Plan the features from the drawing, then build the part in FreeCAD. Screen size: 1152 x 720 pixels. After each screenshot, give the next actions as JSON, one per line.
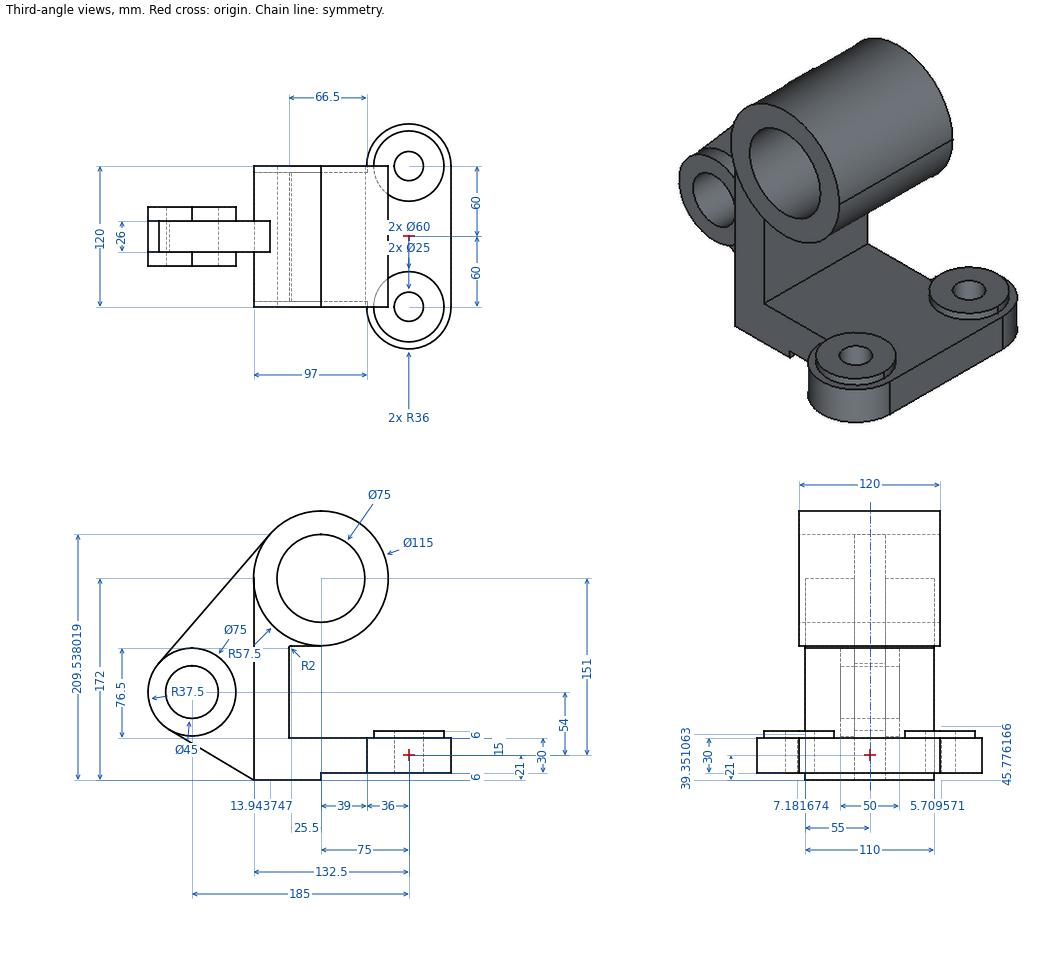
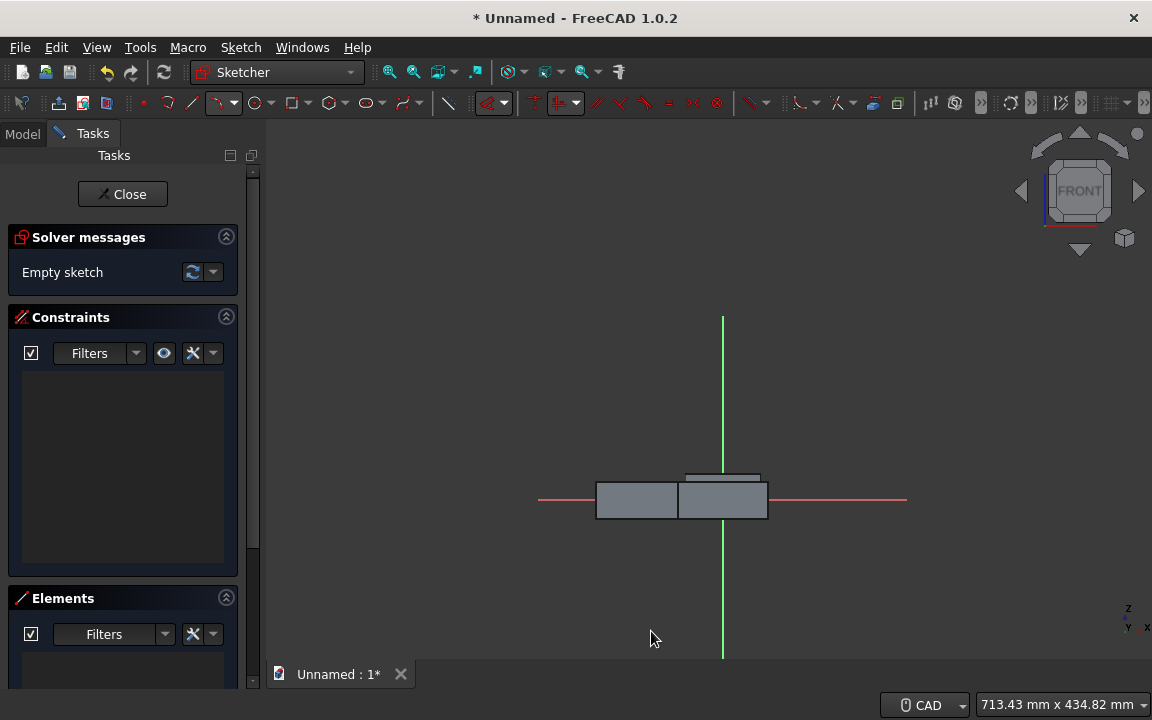
{"action": "left_click", "coordinate": [256, 104]}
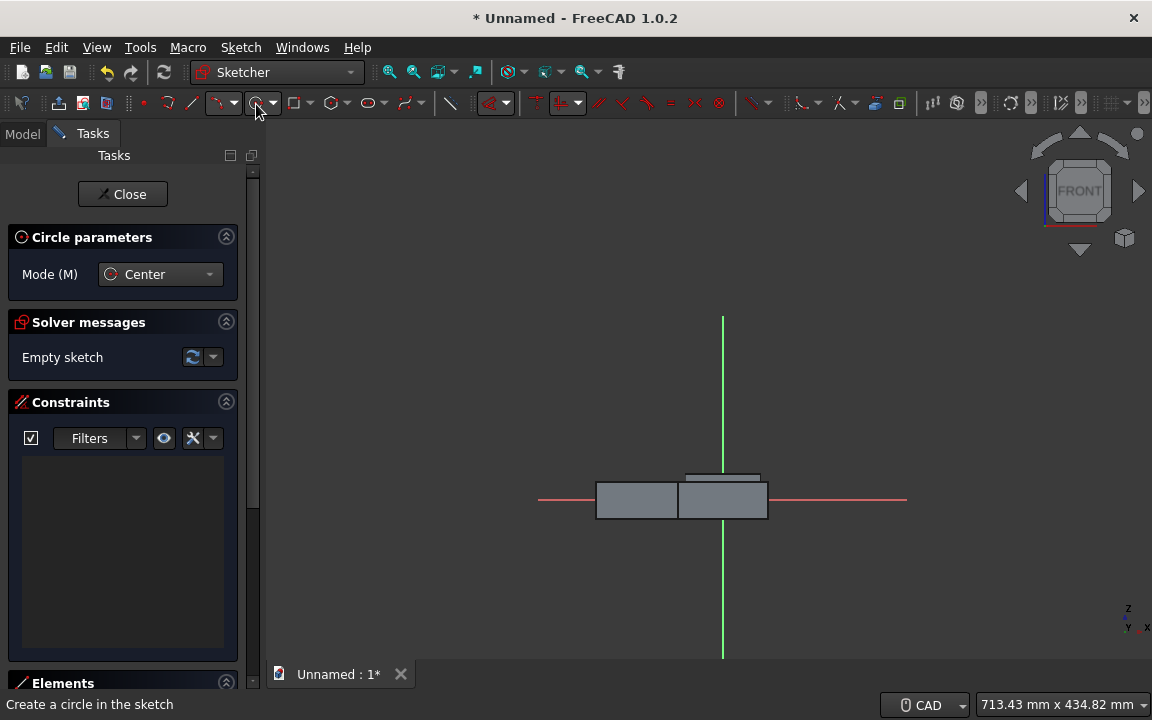
{"action": "left_click", "coordinate": [630, 313]}
{"action": "left_click", "coordinate": [680, 262]}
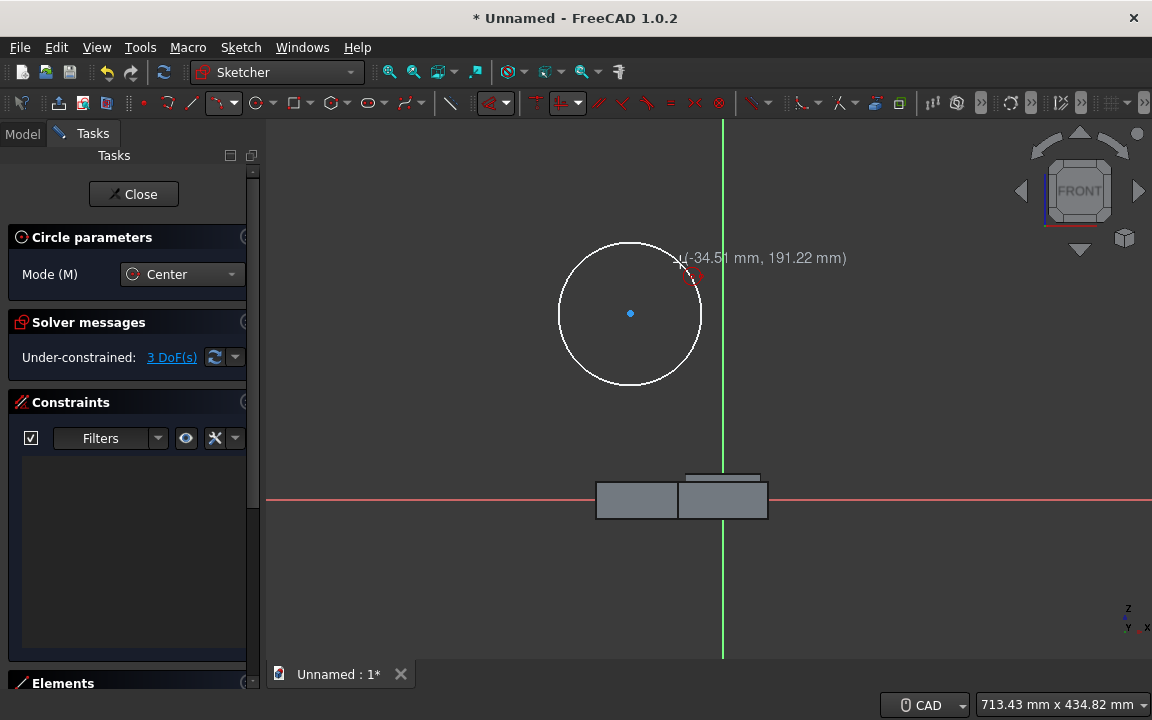
{"action": "left_click", "coordinate": [630, 314]}
{"action": "left_click", "coordinate": [663, 280]}
{"action": "key", "text": "Escape"}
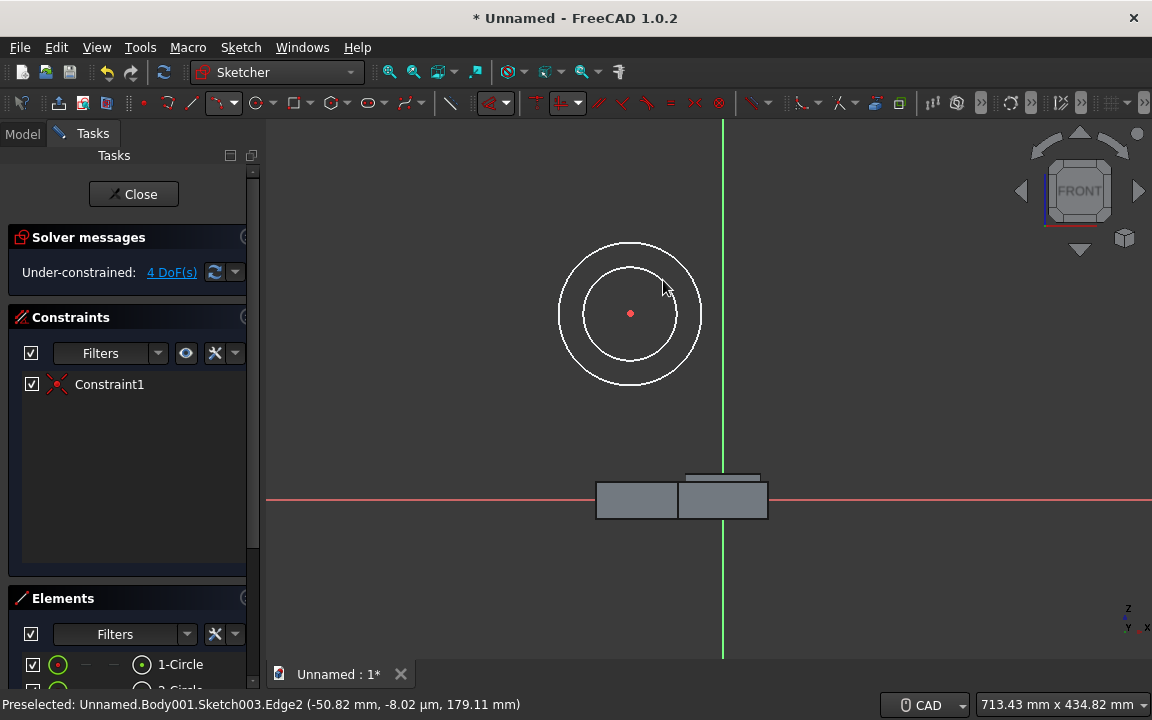
{"action": "left_click", "coordinate": [680, 263]}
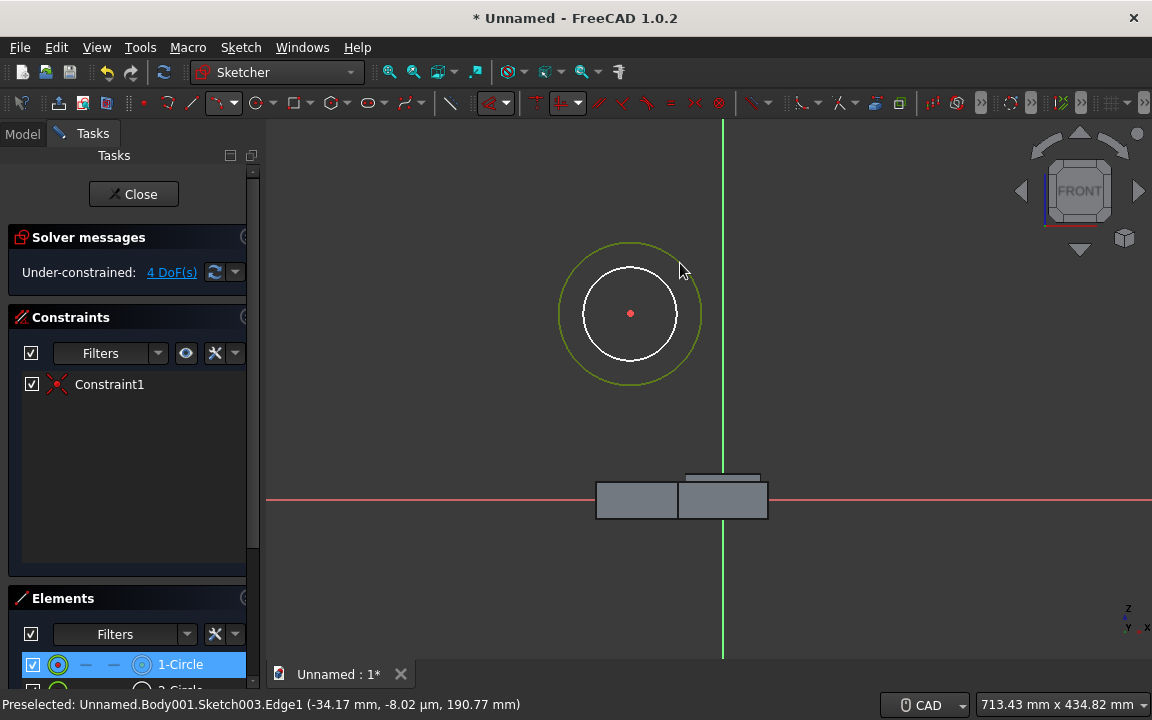
{"action": "key", "text": "k o"}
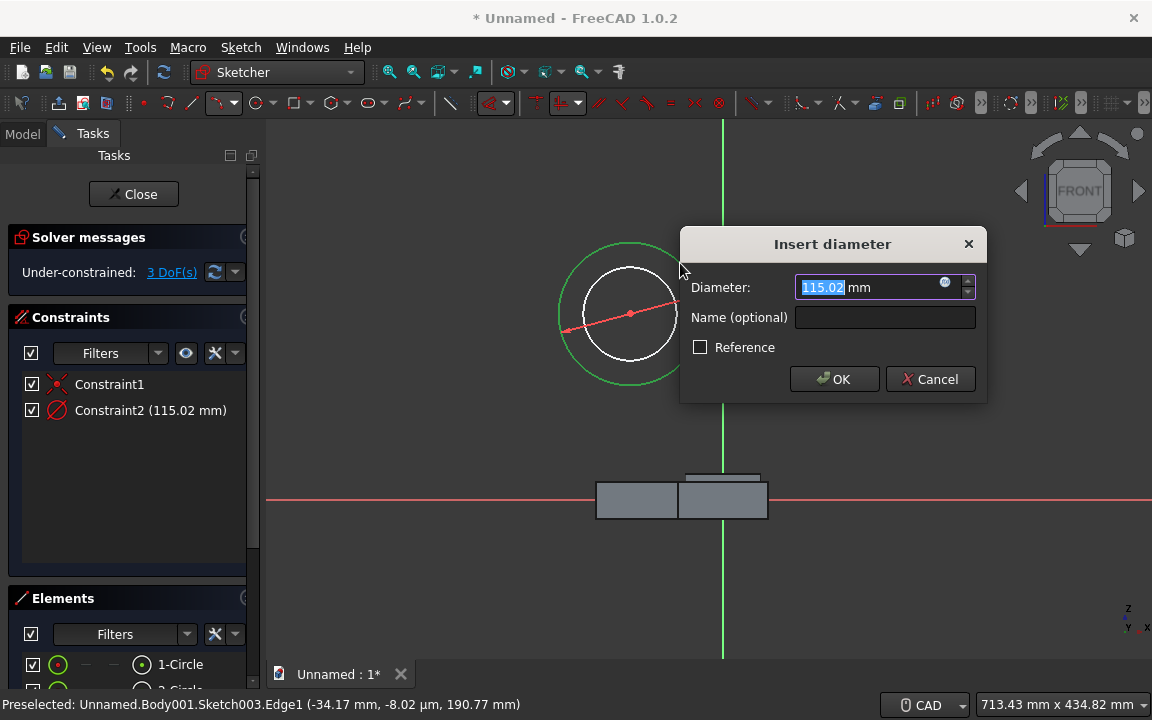
{"action": "type", "text": "115"}
{"action": "key", "text": "Return"}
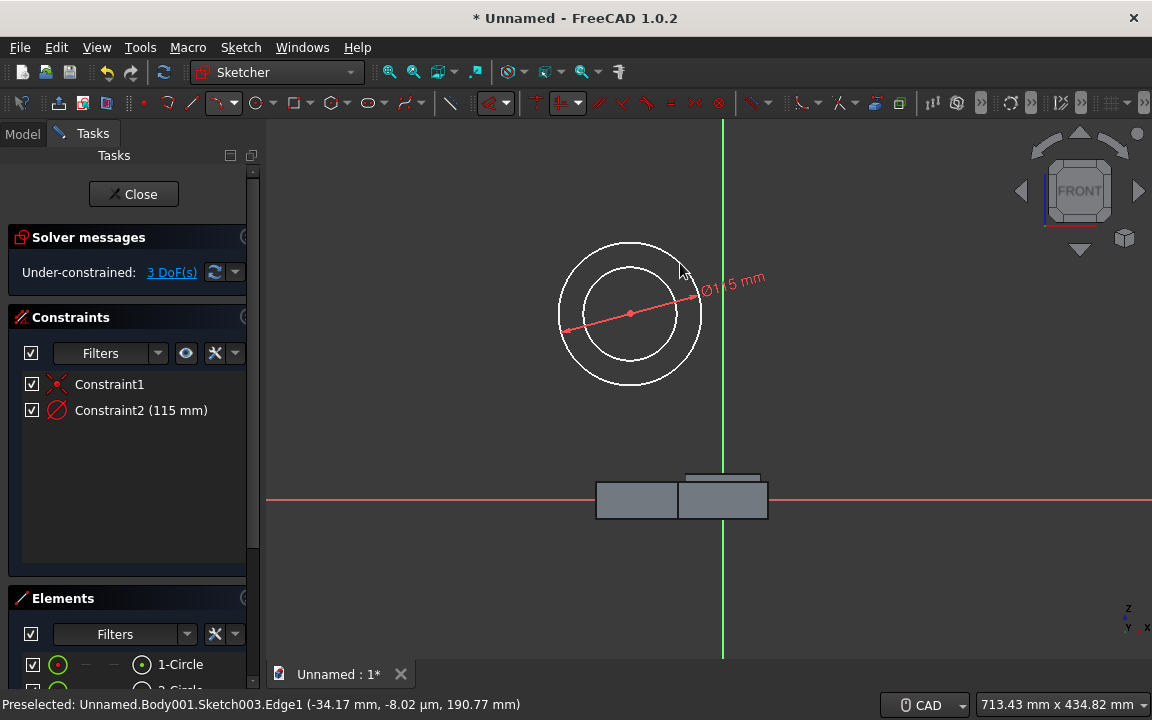
{"action": "left_click", "coordinate": [663, 281]}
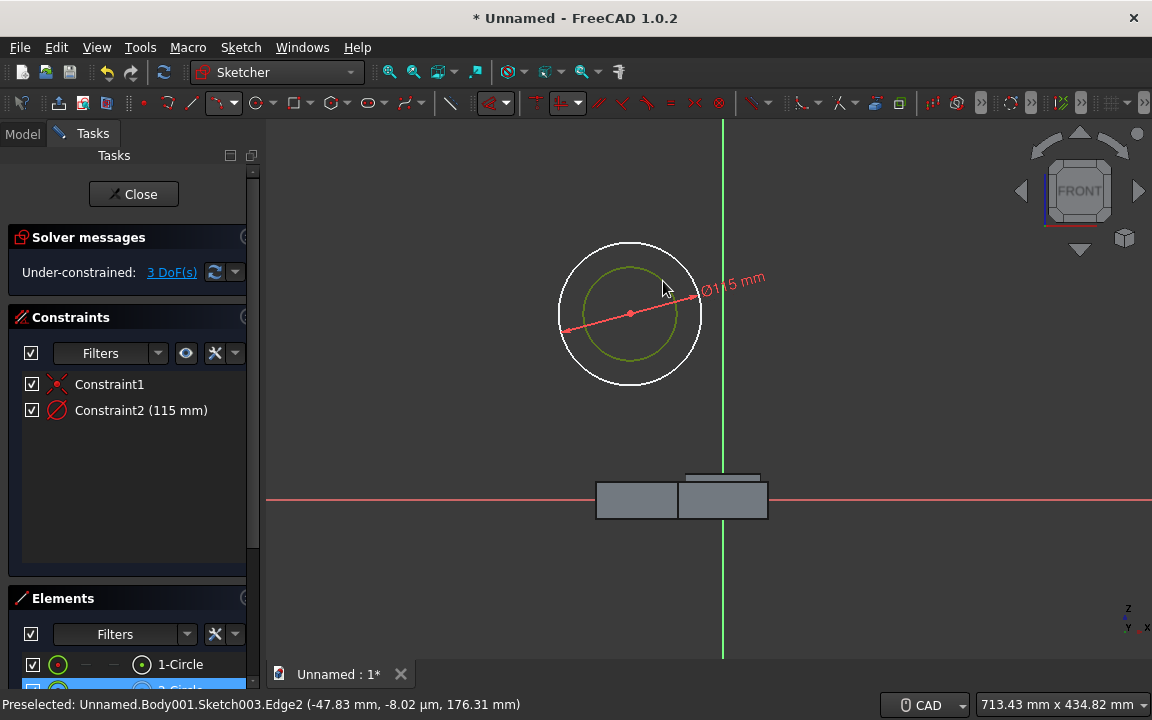
{"action": "key", "text": "k o"}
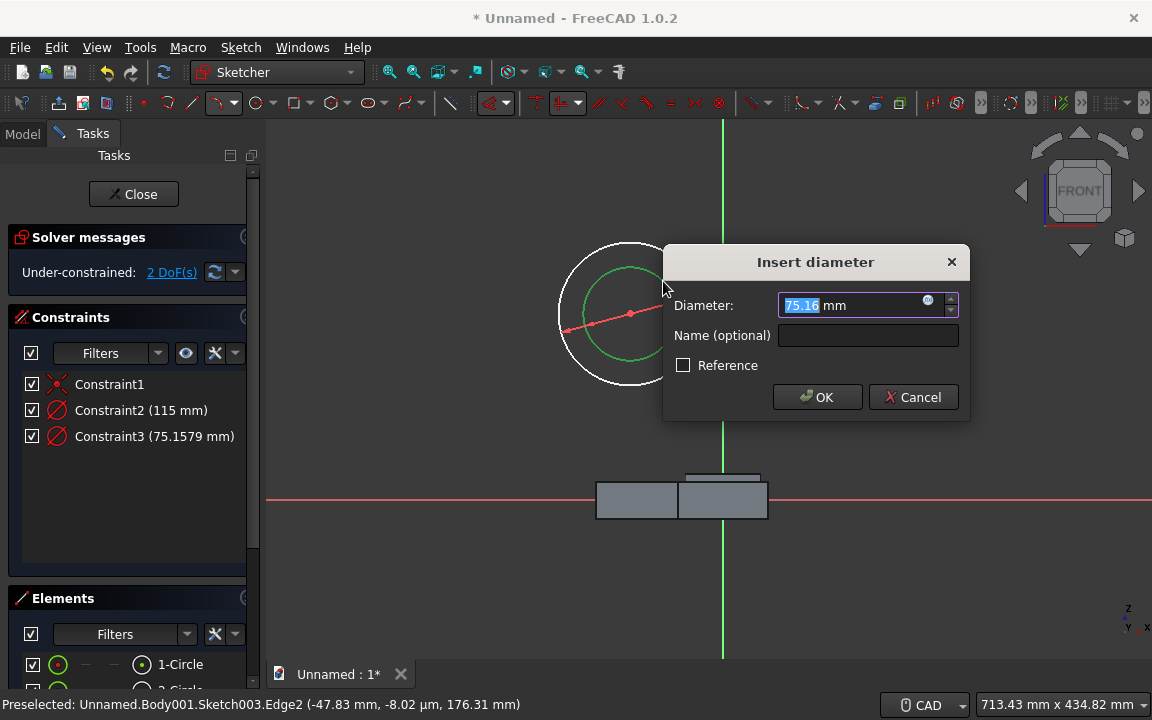
{"action": "type", "text": "75"}
{"action": "key", "text": "Return"}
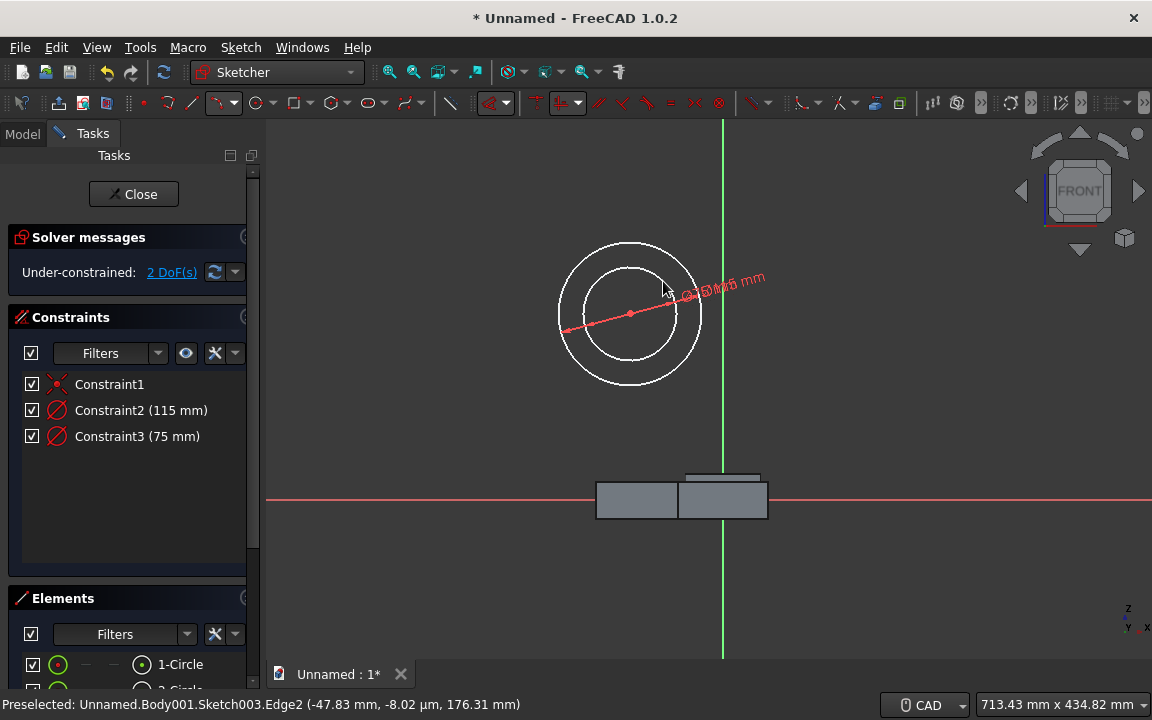
{"action": "left_click", "coordinate": [630, 314]}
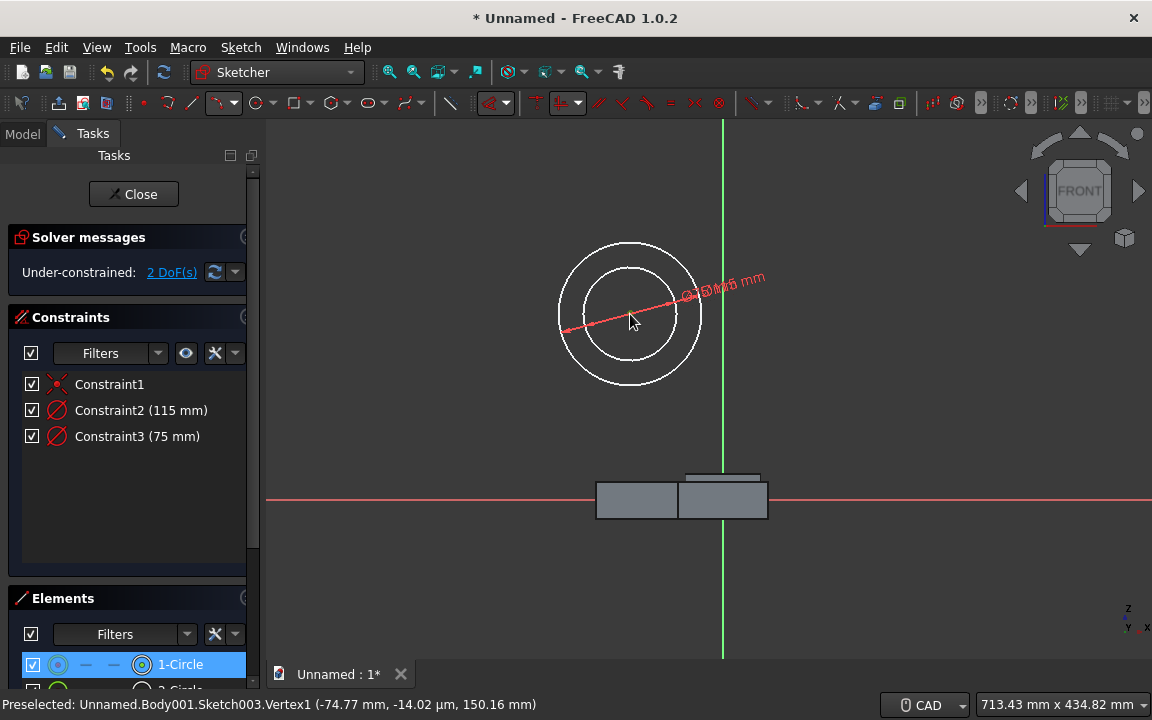
{"action": "key", "text": "l"}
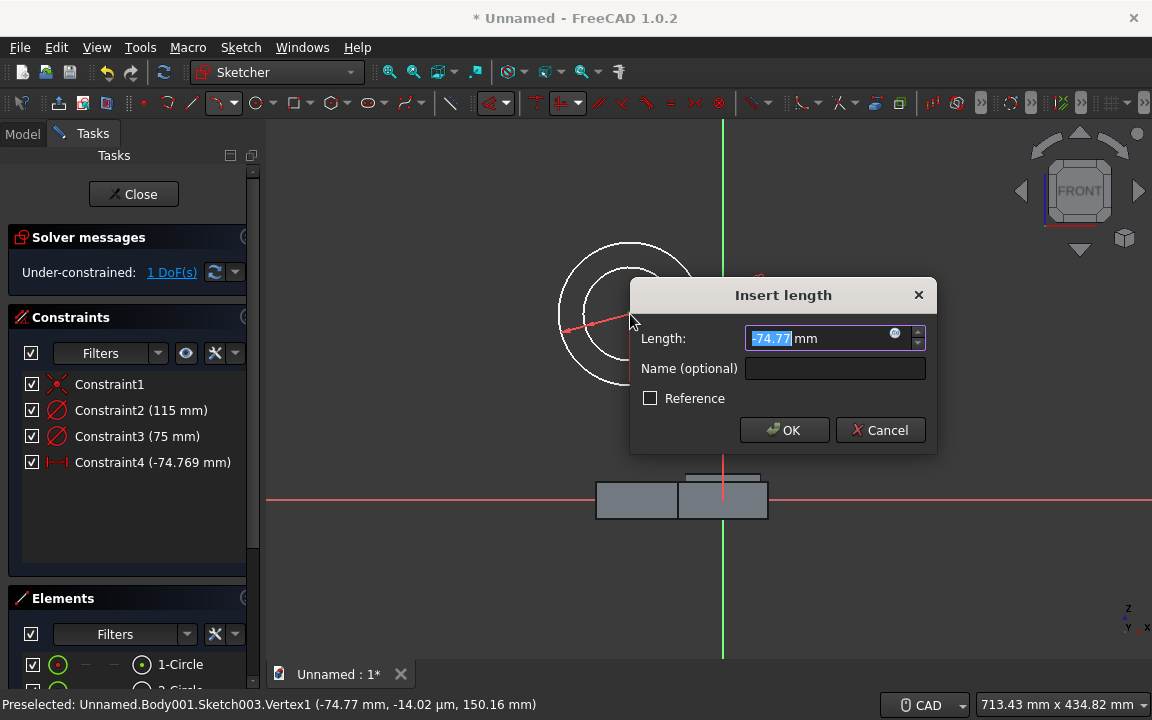
{"action": "type", "text": "-75"}
{"action": "key", "text": "Return"}